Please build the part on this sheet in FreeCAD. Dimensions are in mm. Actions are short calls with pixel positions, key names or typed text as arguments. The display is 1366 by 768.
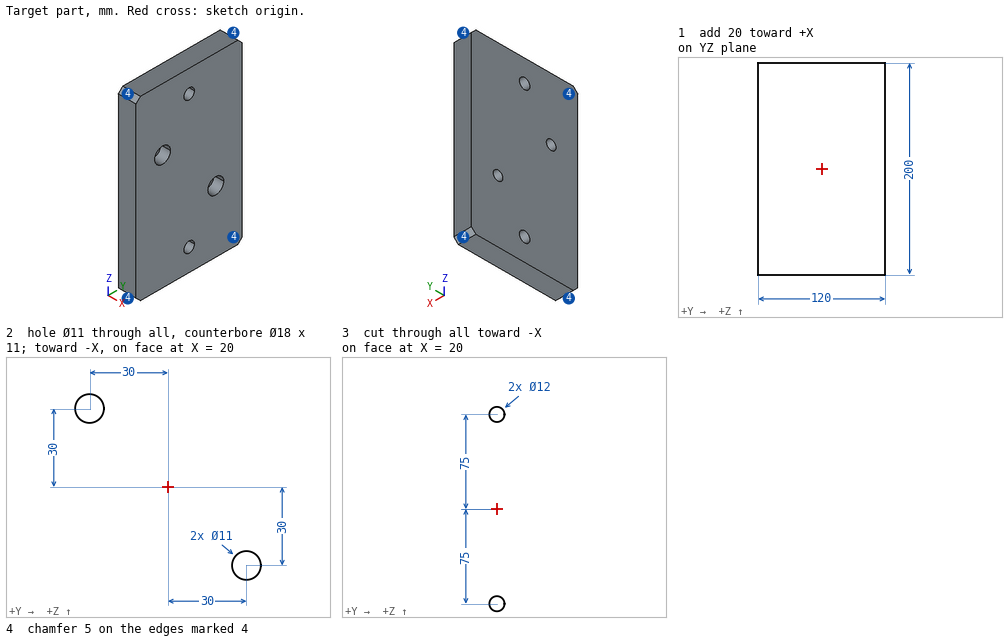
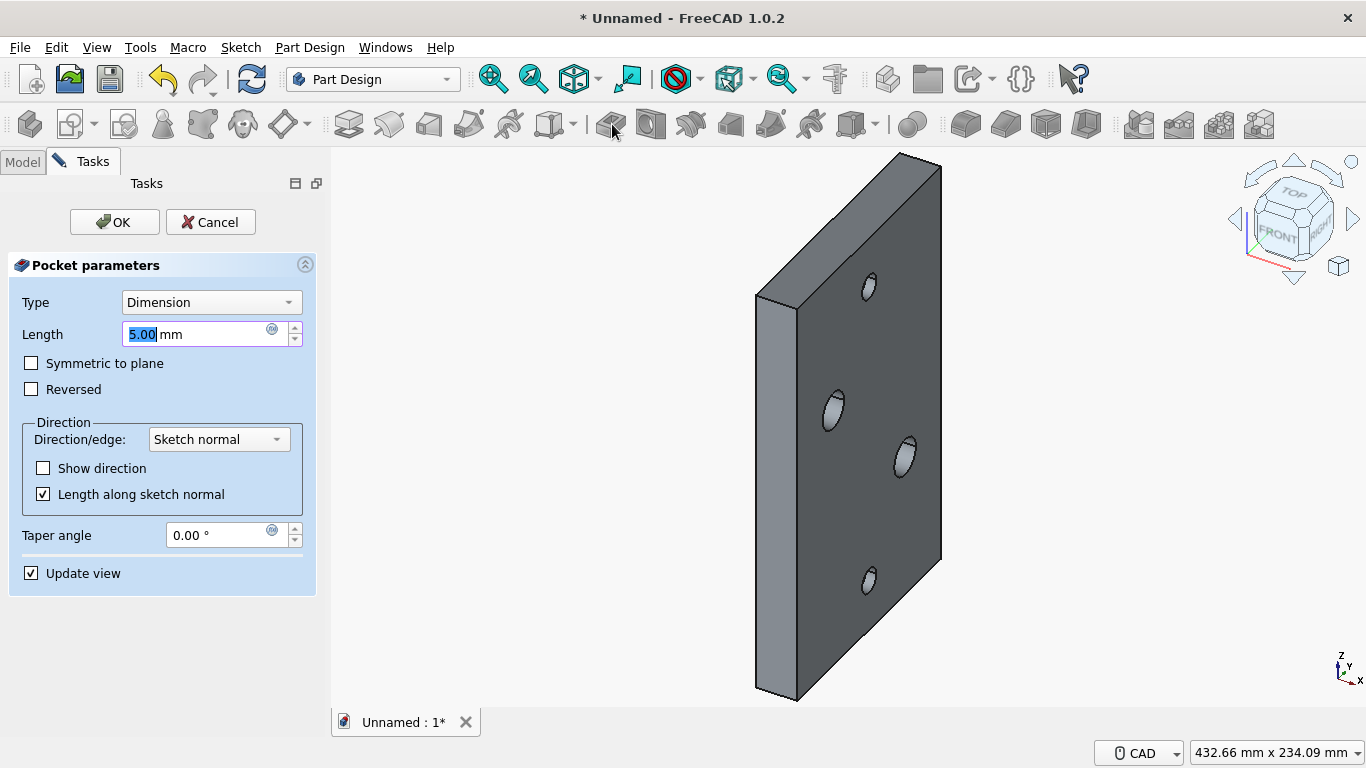
click(212, 302)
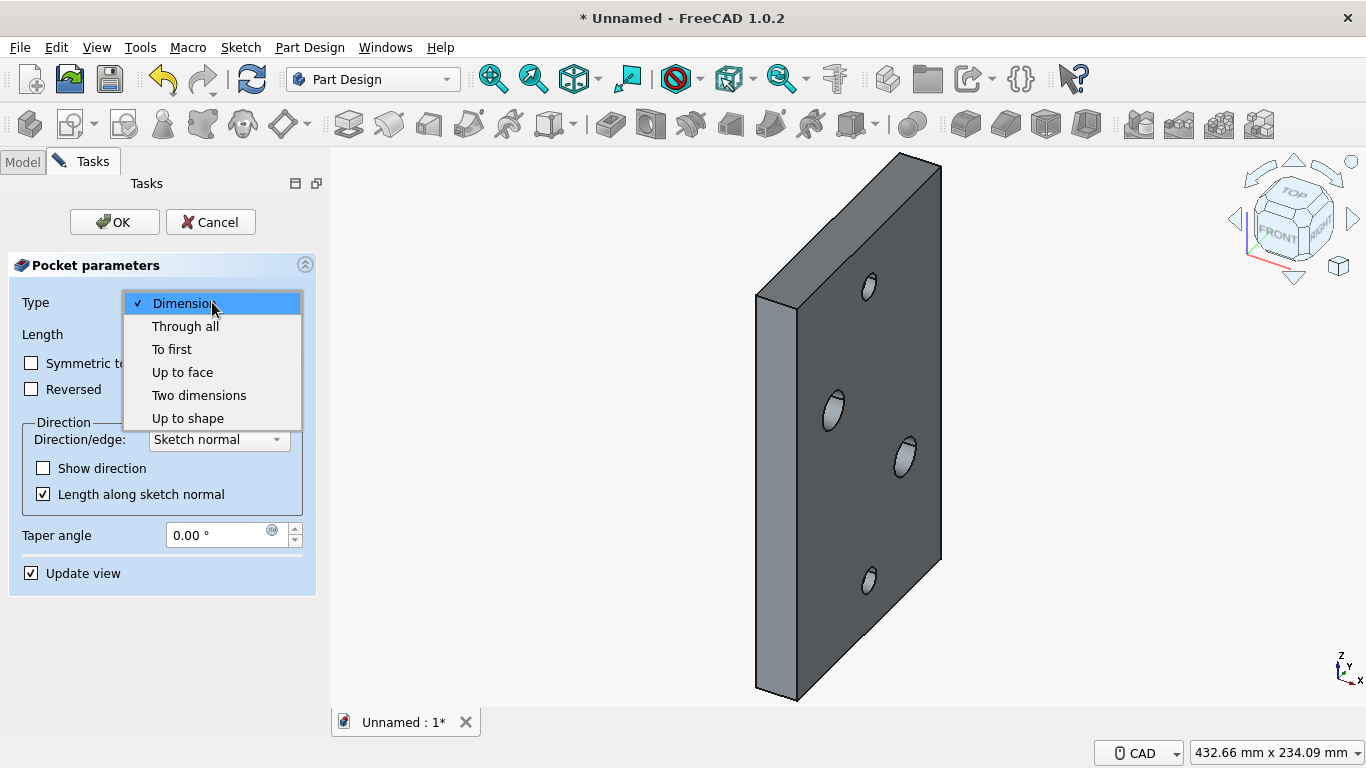
click(212, 326)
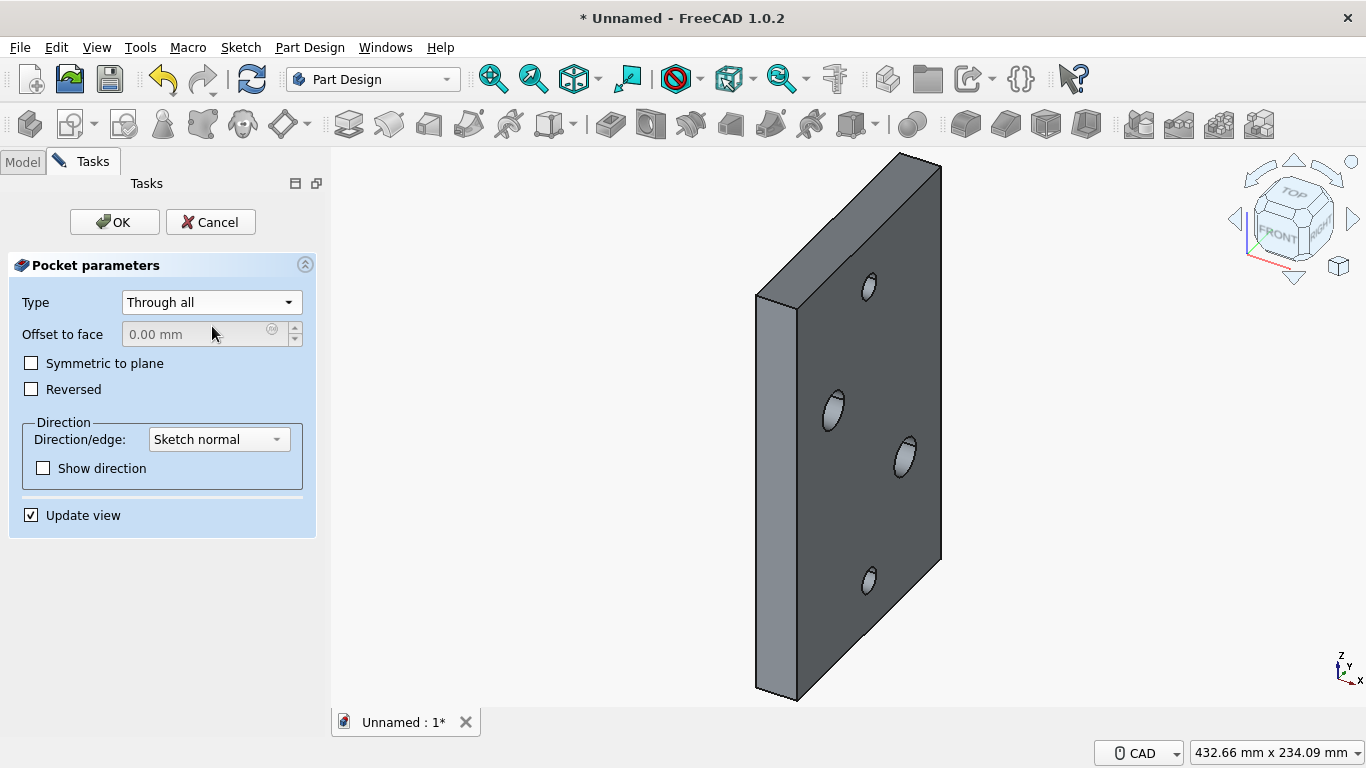
click(115, 222)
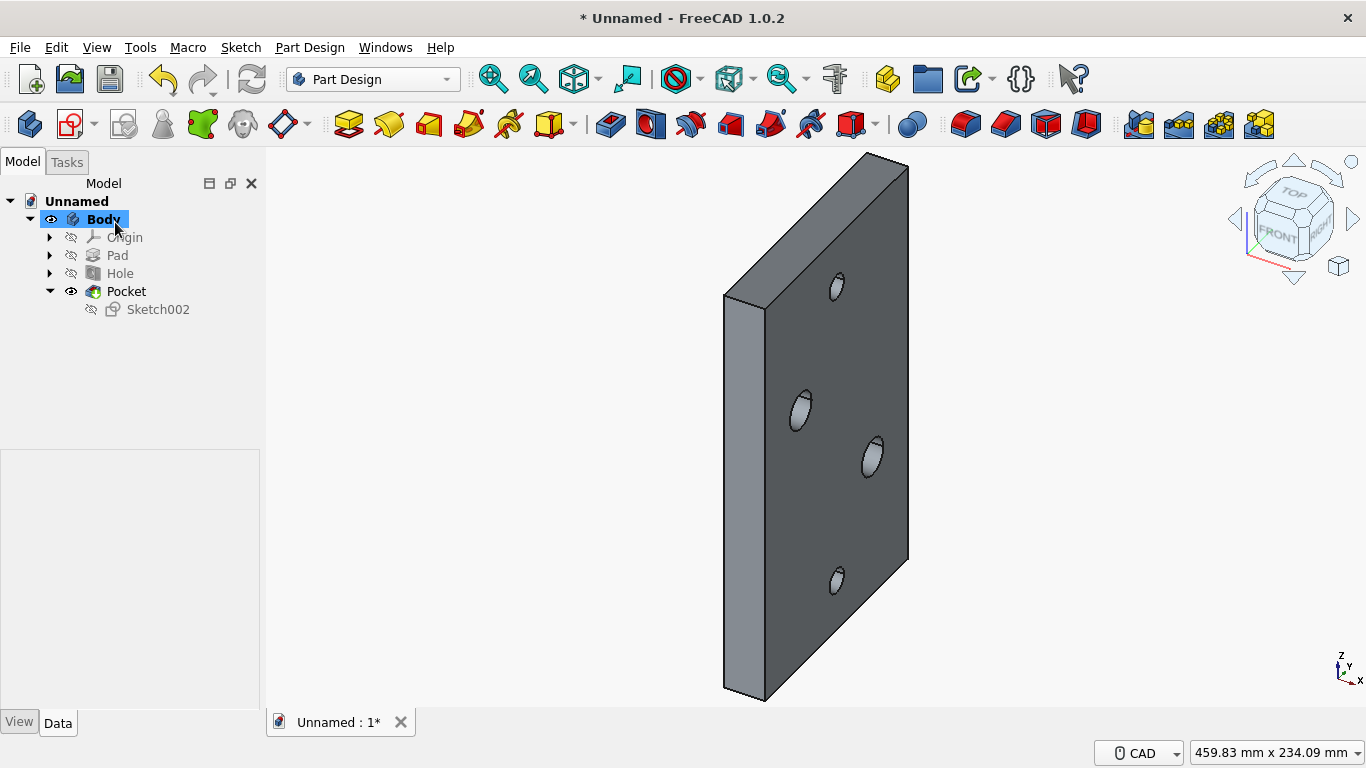
click(744, 301)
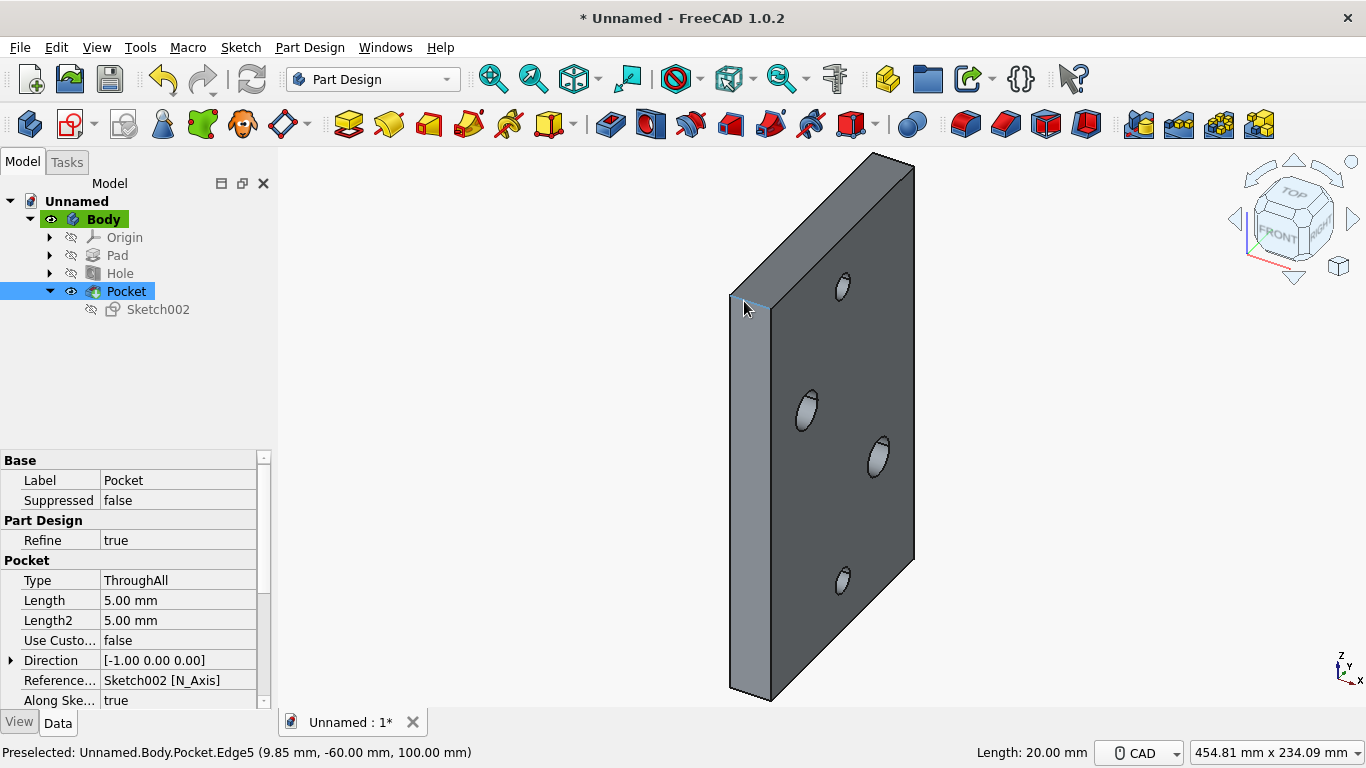
key(0)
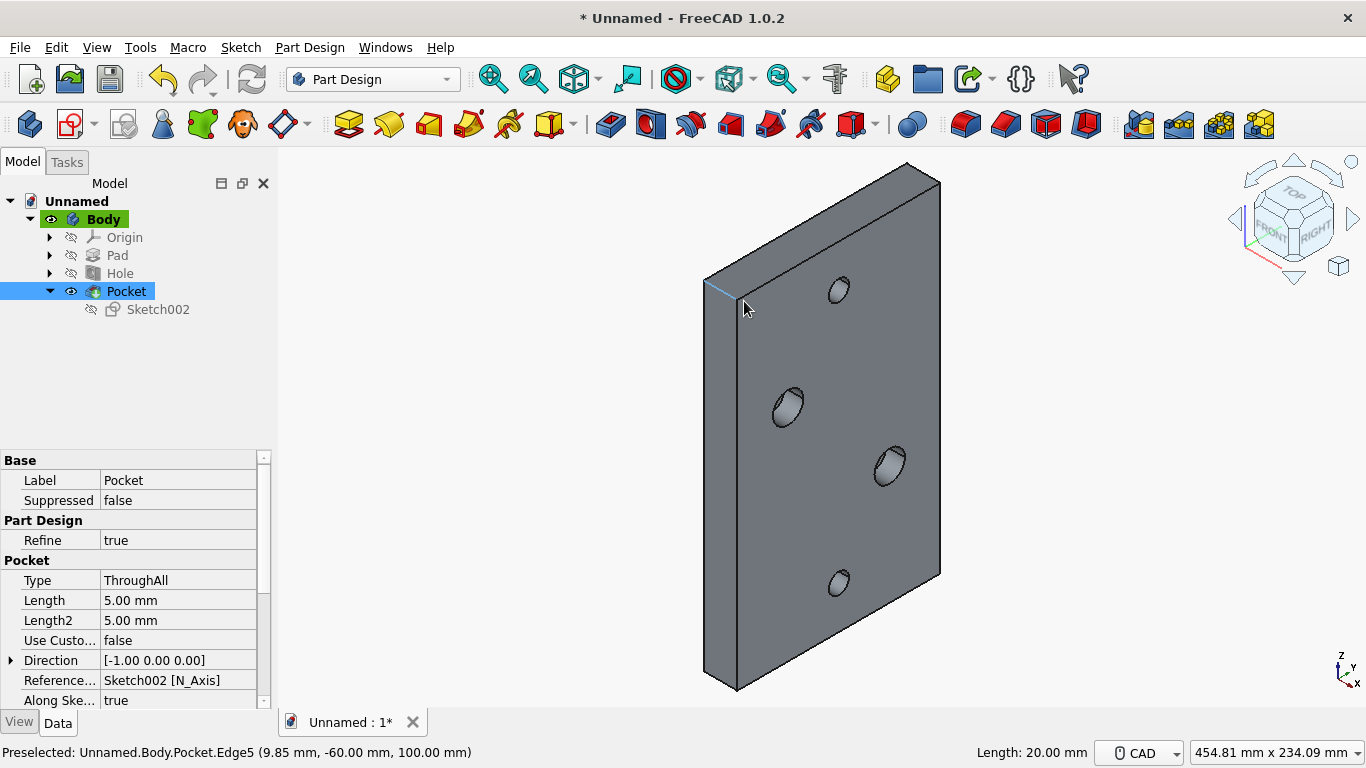
key(2)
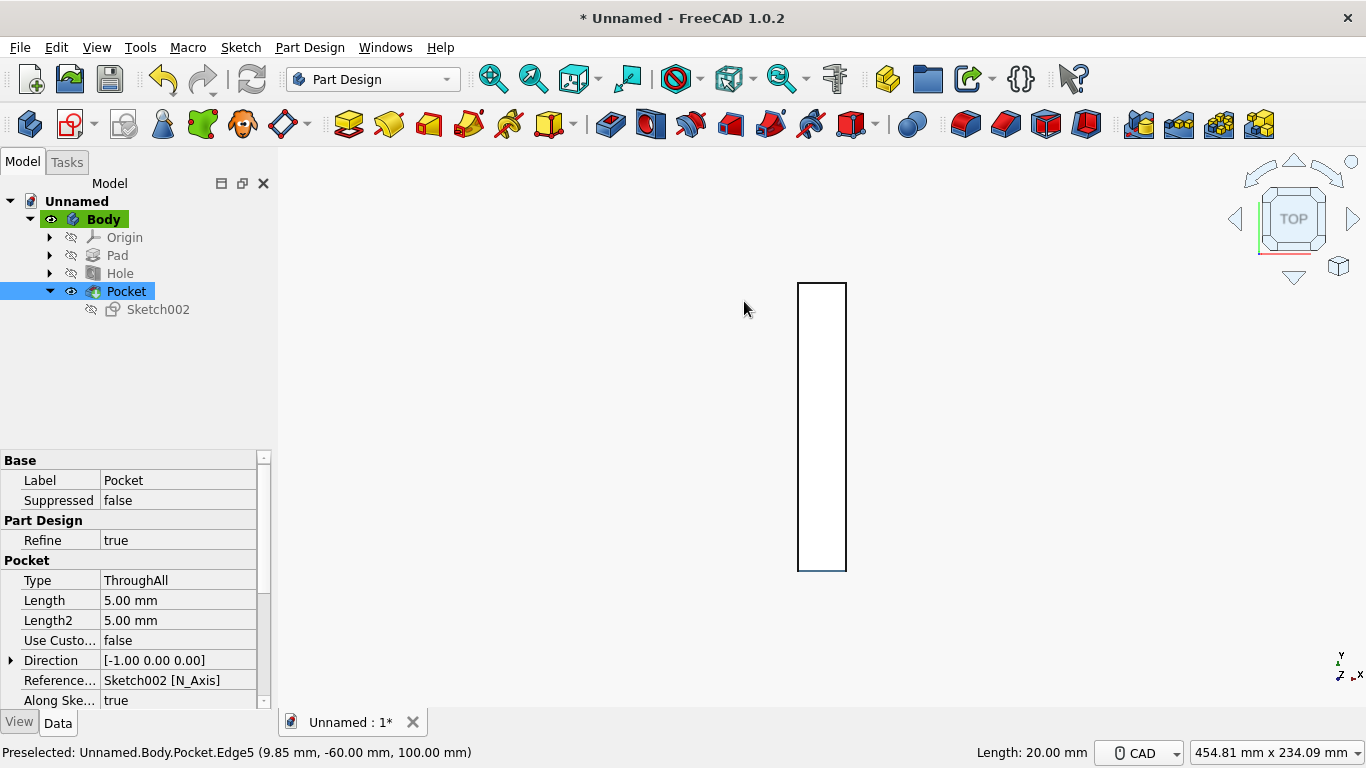
click(822, 282, ctrl)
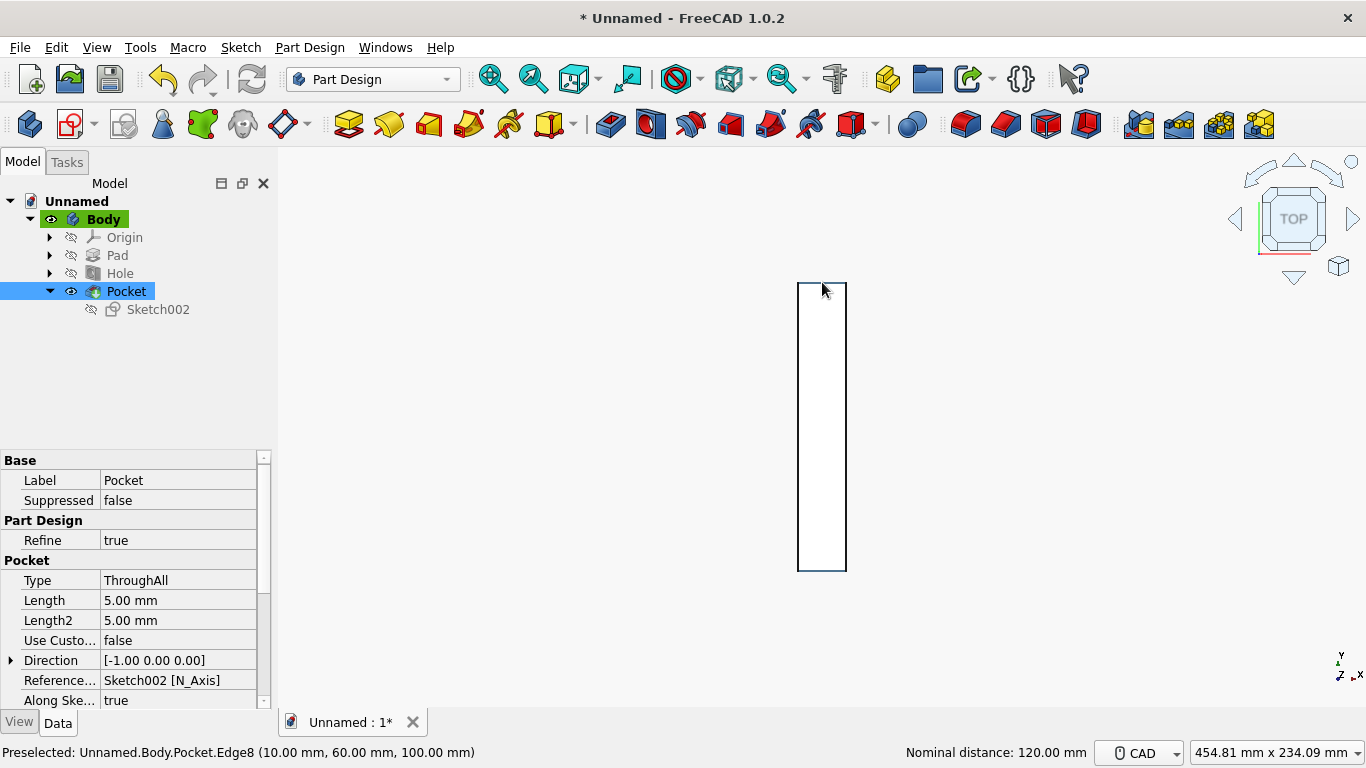
key(1)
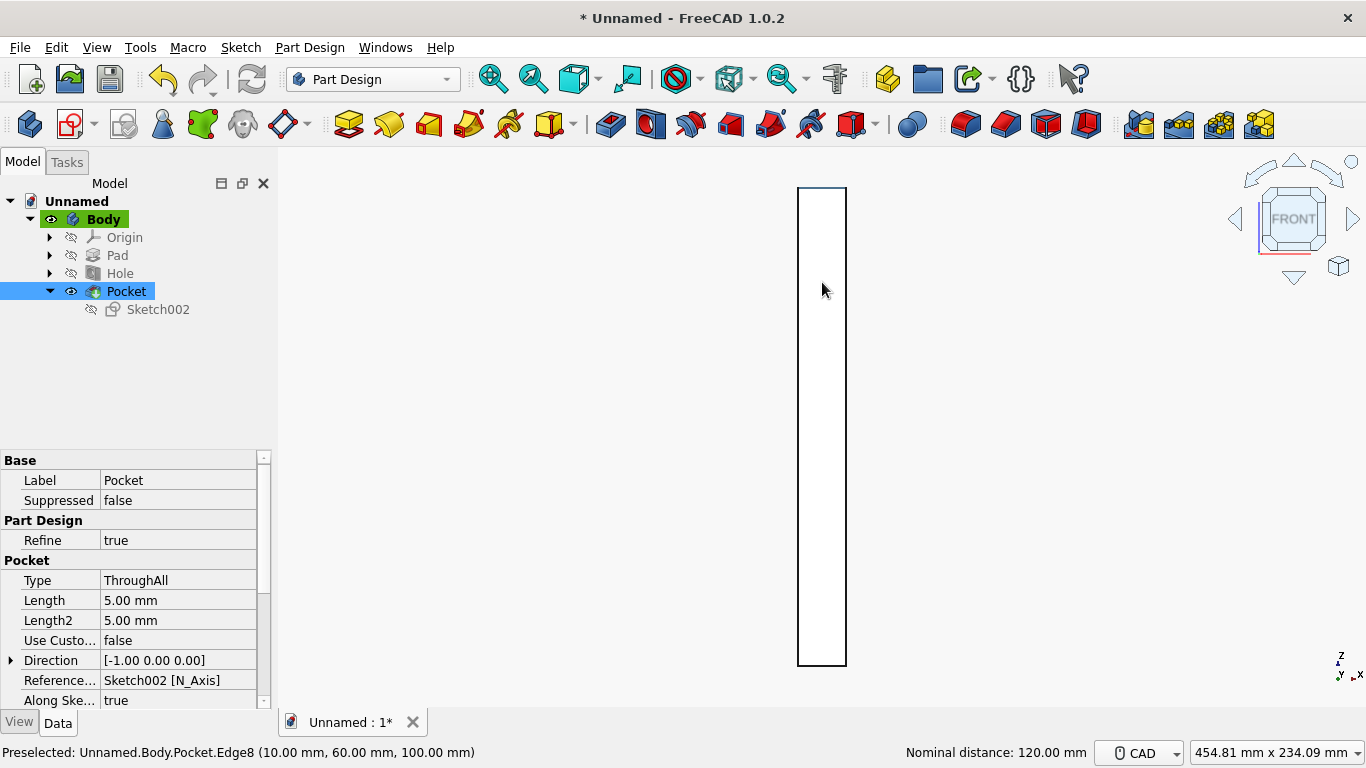
click(822, 665, ctrl)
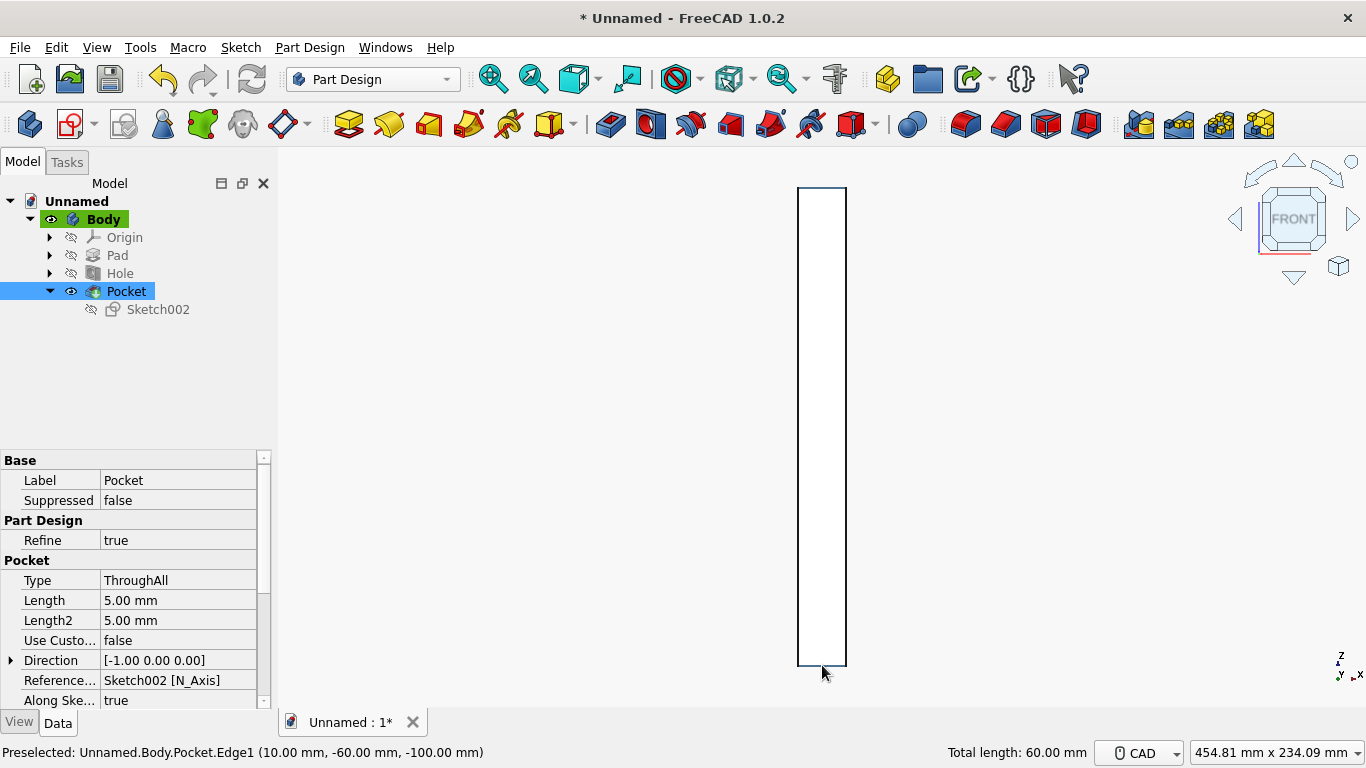
key(3)